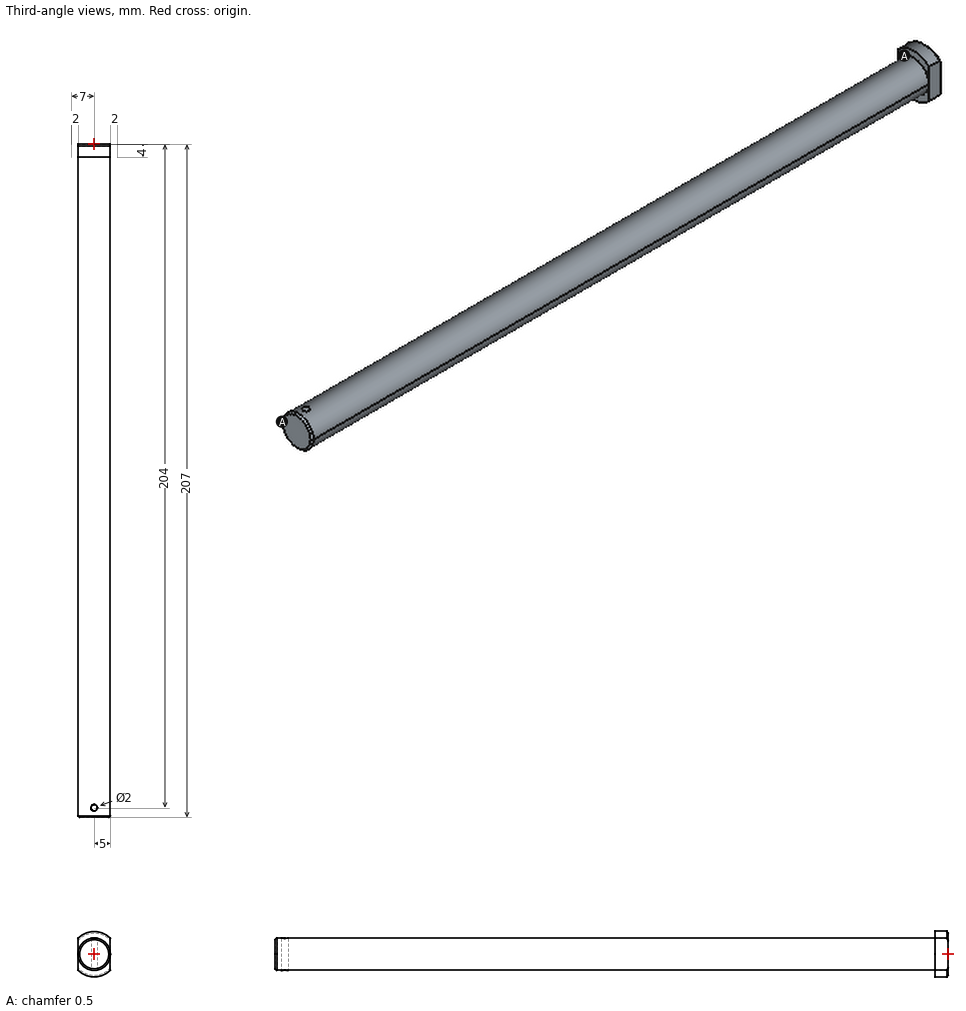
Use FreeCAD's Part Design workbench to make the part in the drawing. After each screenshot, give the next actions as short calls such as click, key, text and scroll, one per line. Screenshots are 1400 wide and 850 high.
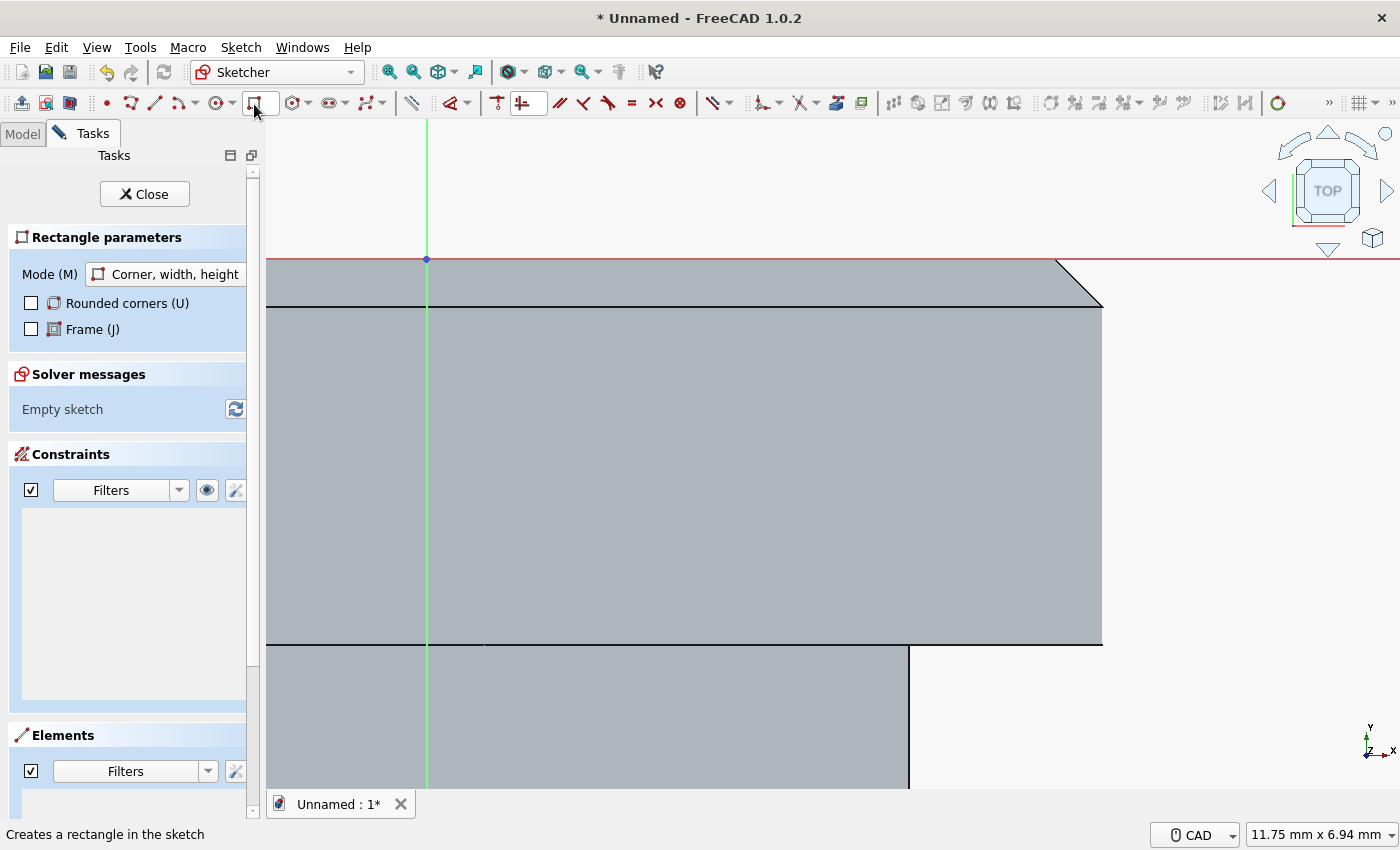
click(909, 259)
click(1102, 645)
key(Escape)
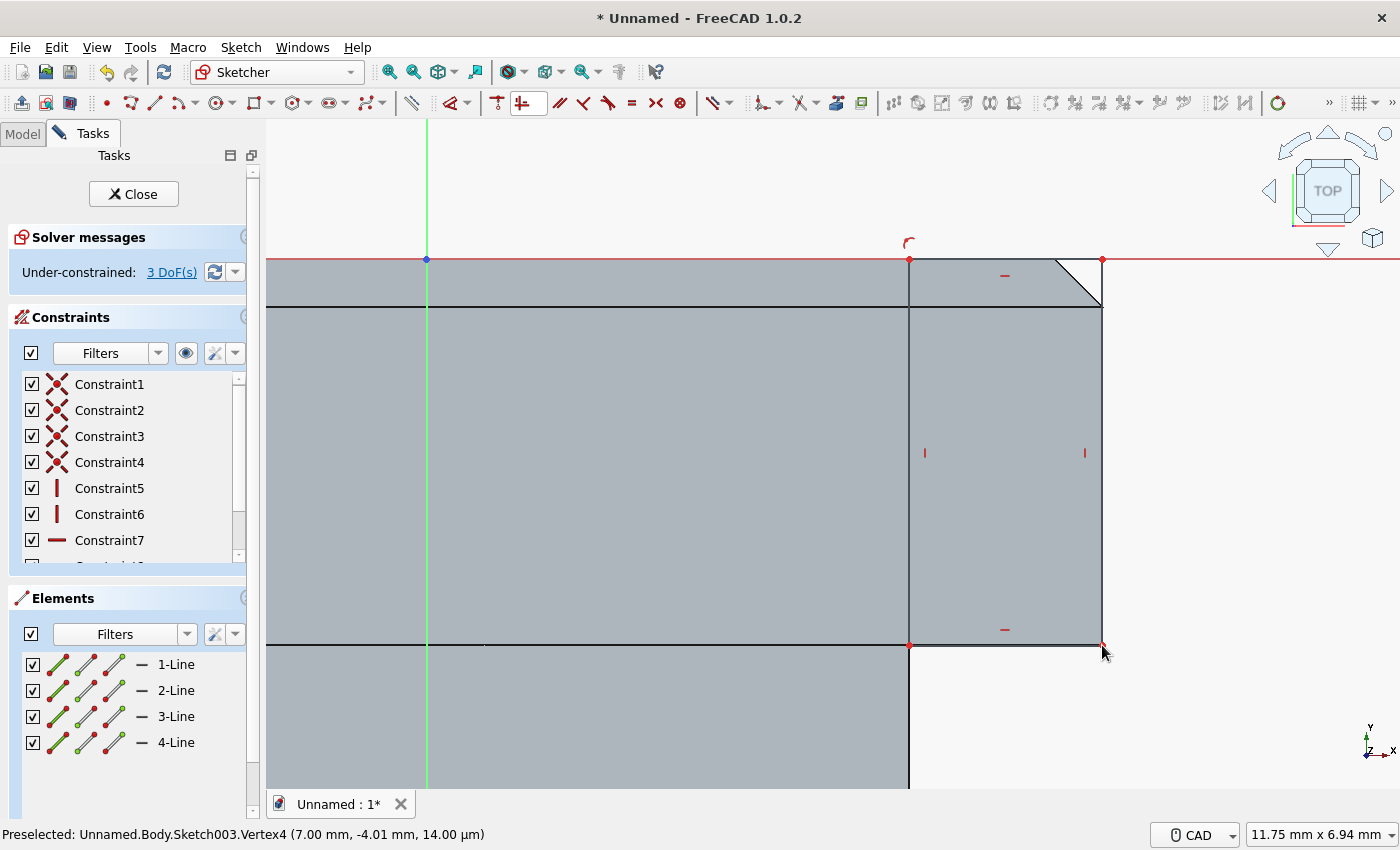
click(450, 104)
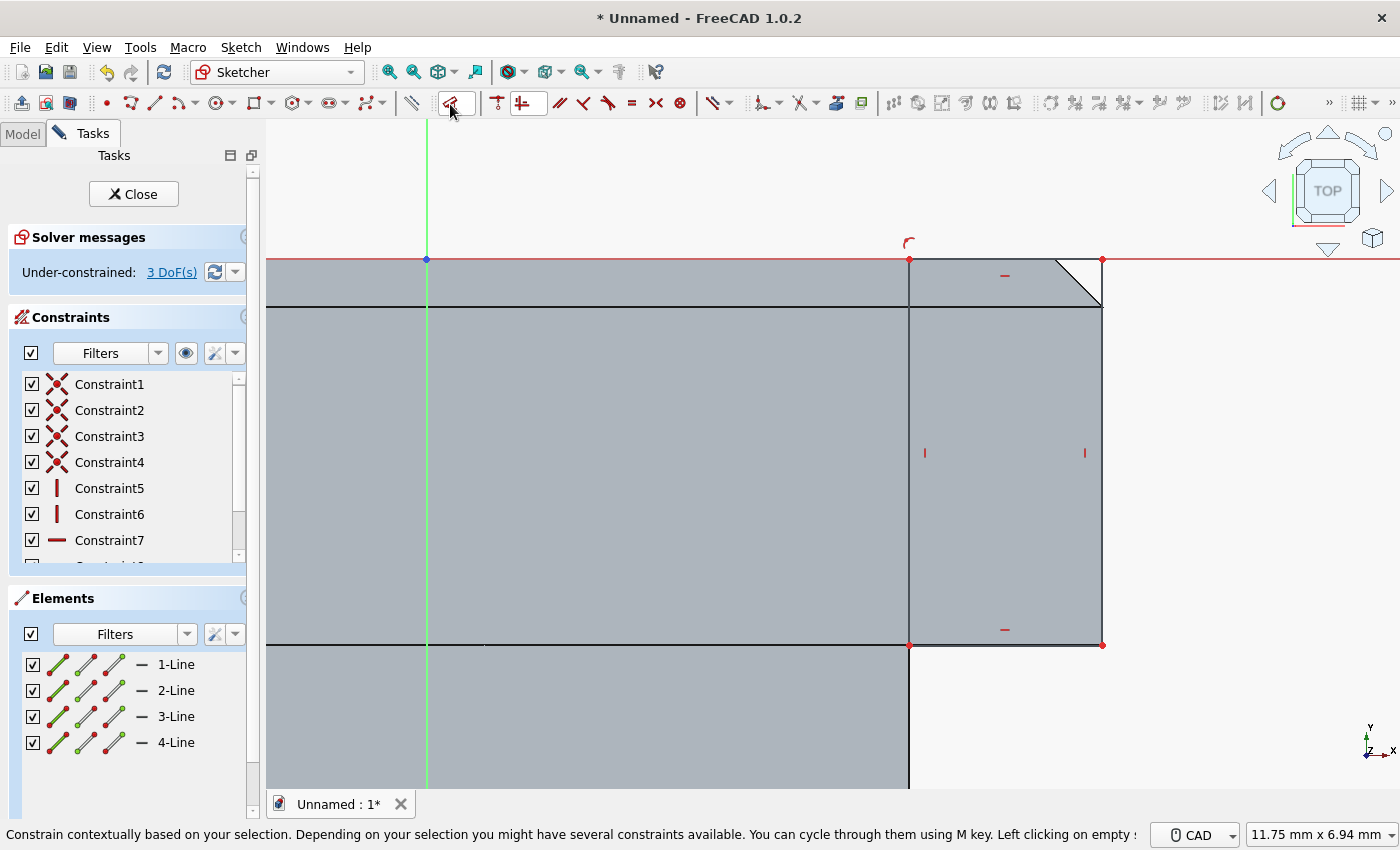
click(909, 375)
click(943, 453)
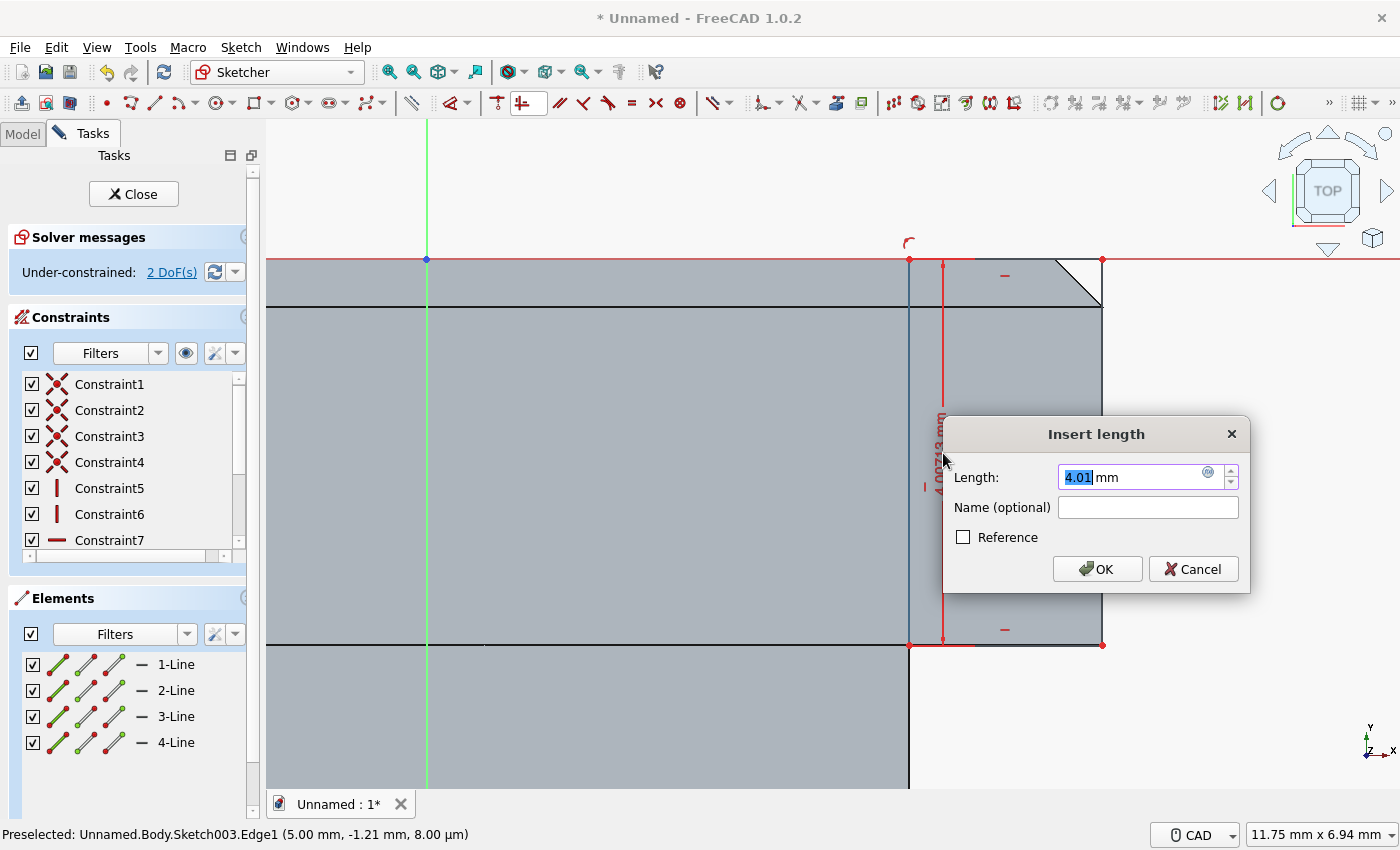
text(4)
key(Return)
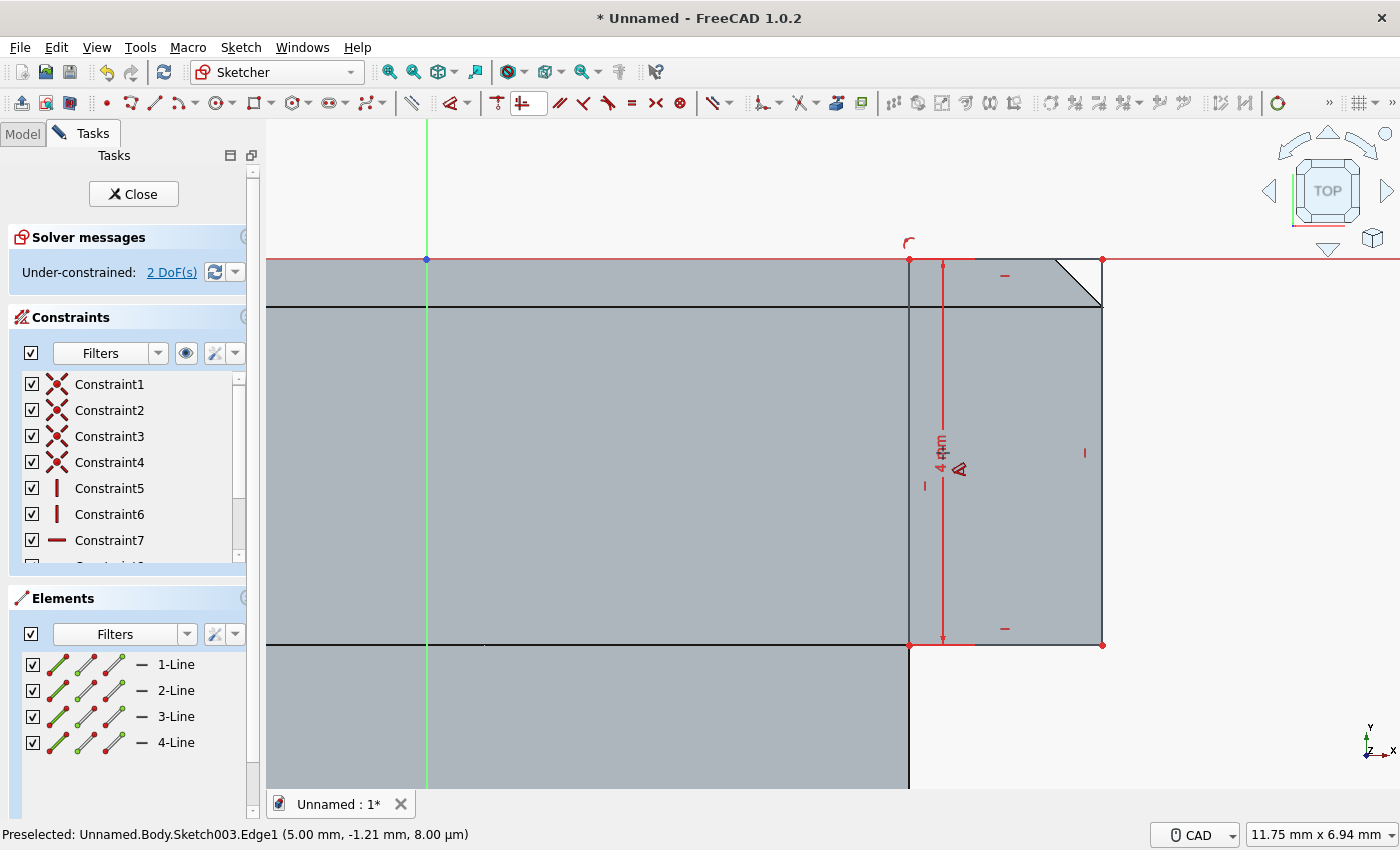
click(967, 645)
click(1006, 679)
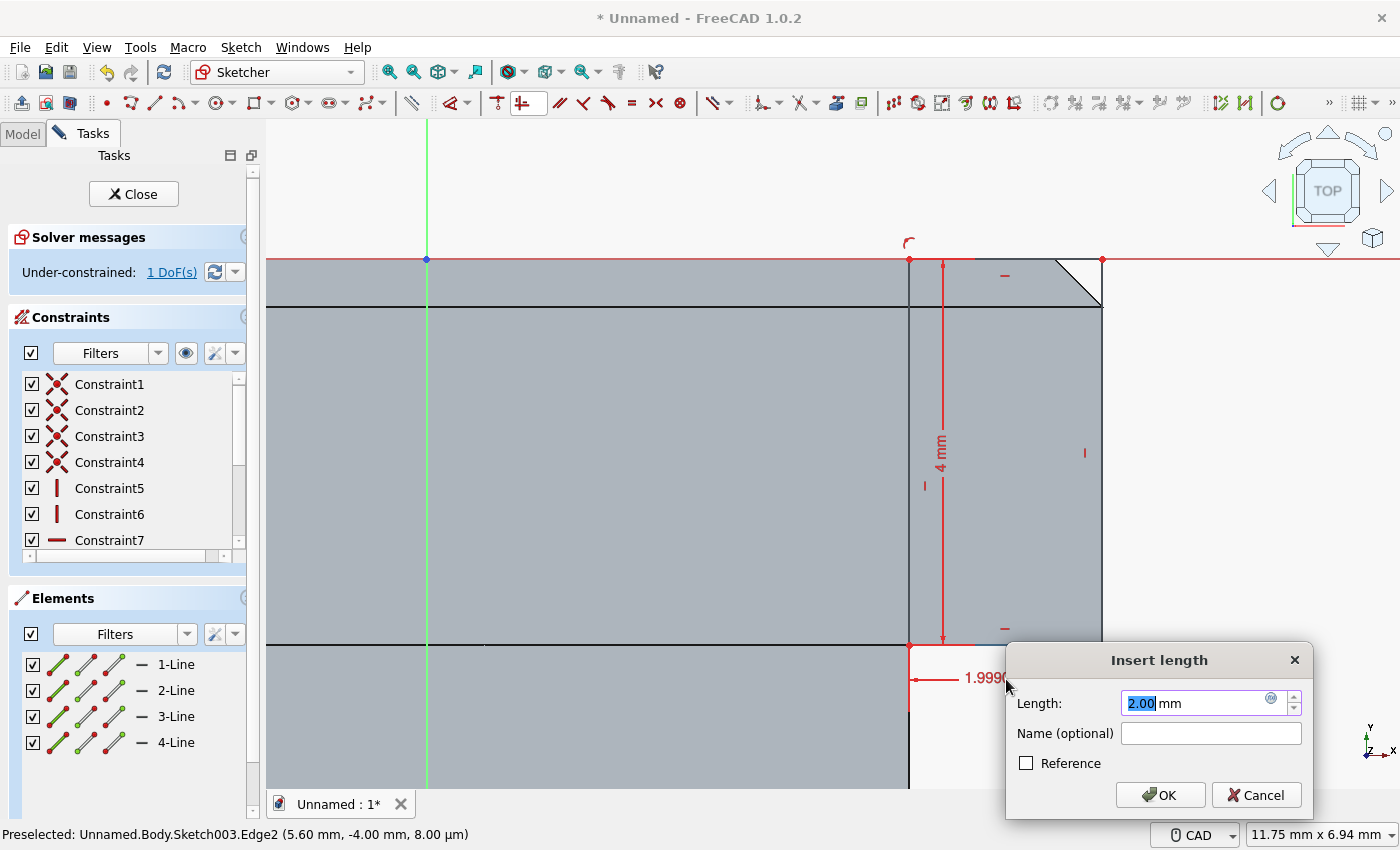
text(2)
key(Return)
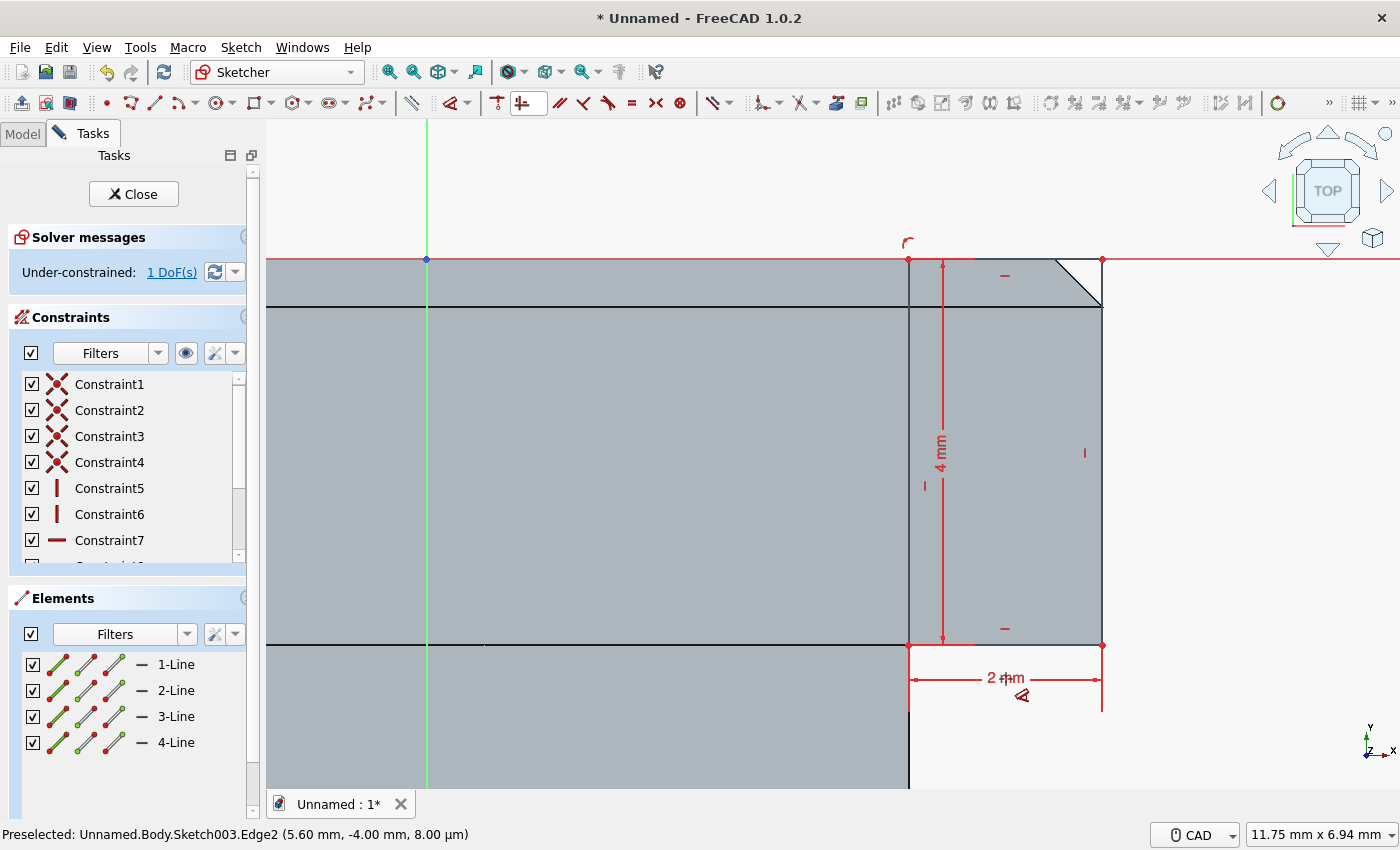
click(909, 259)
click(668, 225)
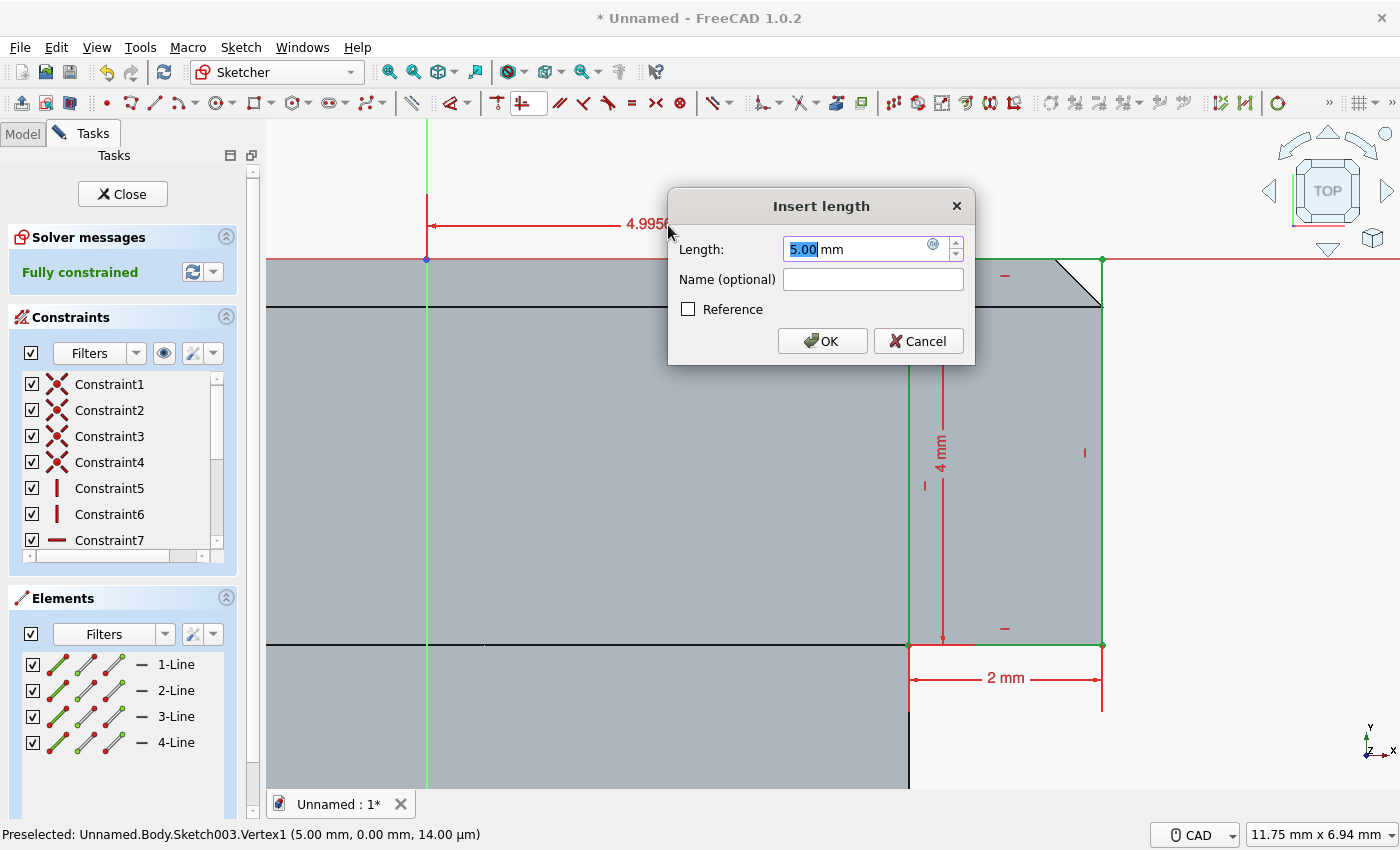
text(5)
key(Return)
key(Escape)